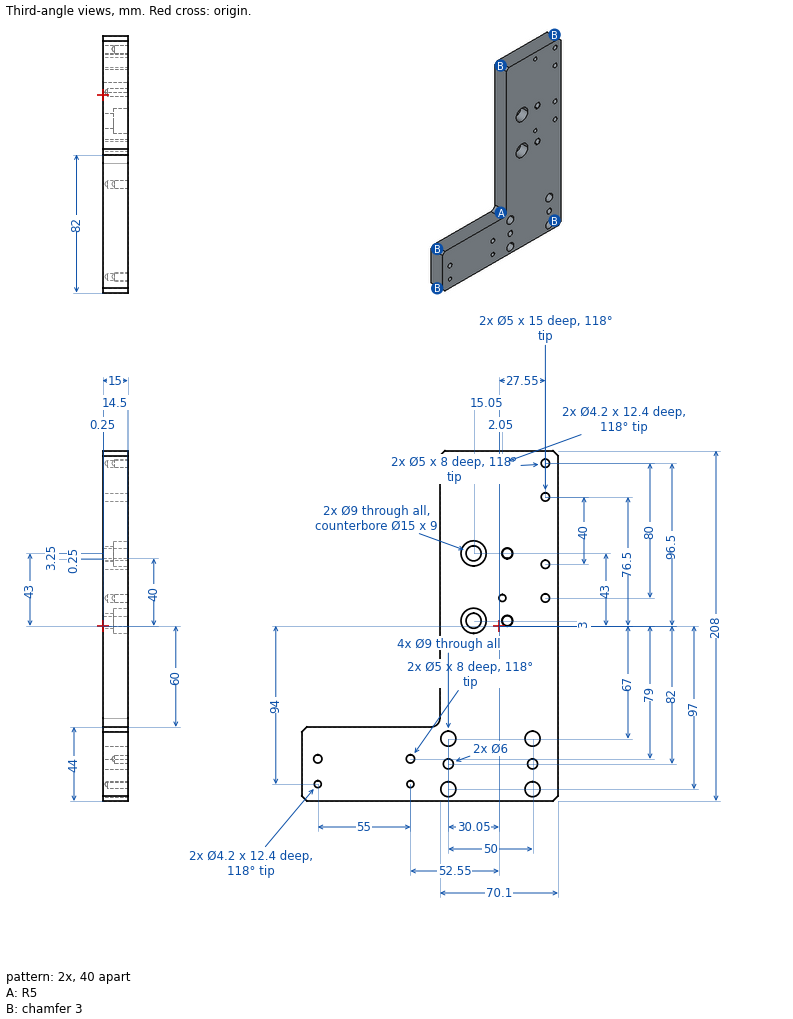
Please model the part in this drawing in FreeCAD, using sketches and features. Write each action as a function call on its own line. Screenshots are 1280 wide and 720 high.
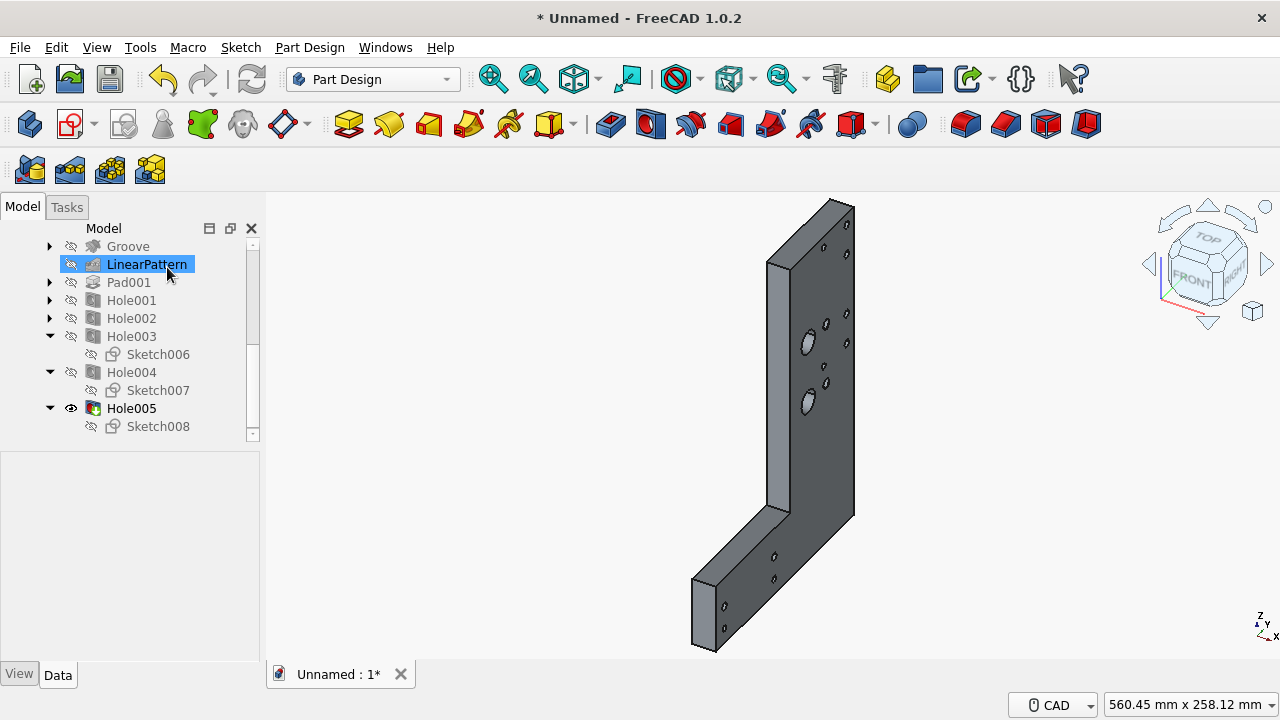
click(824, 477)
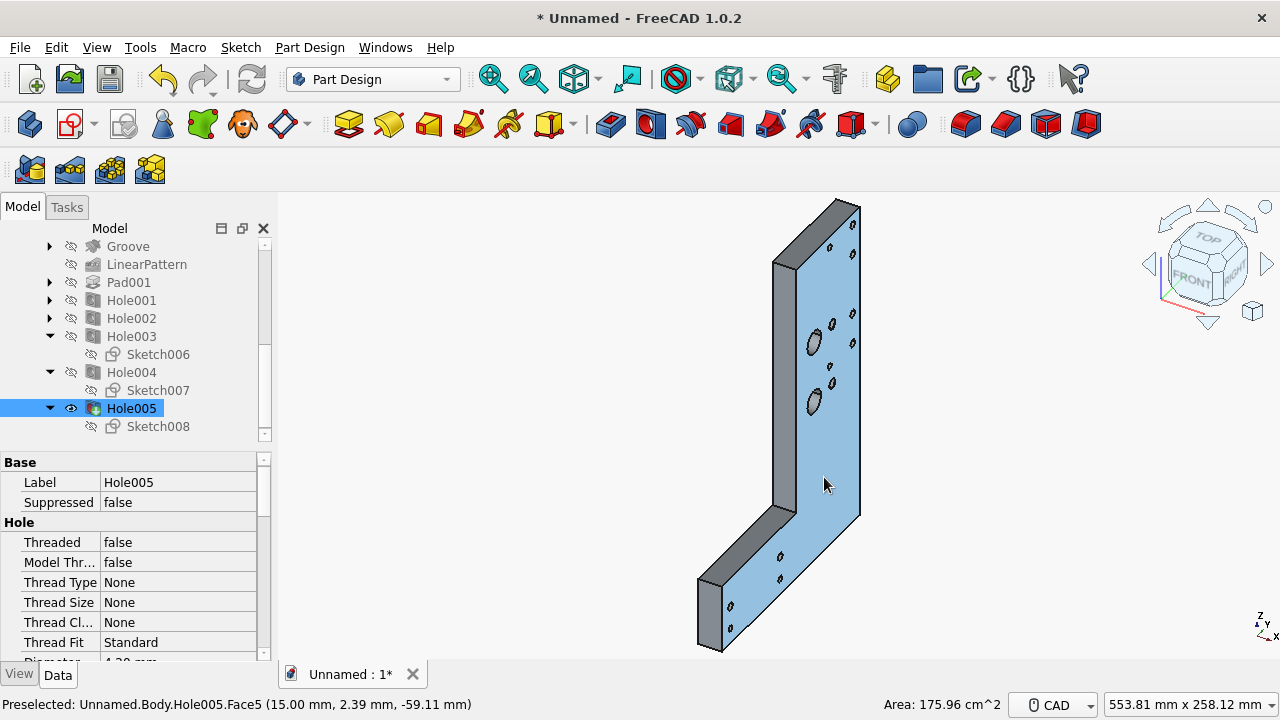
click(70, 124)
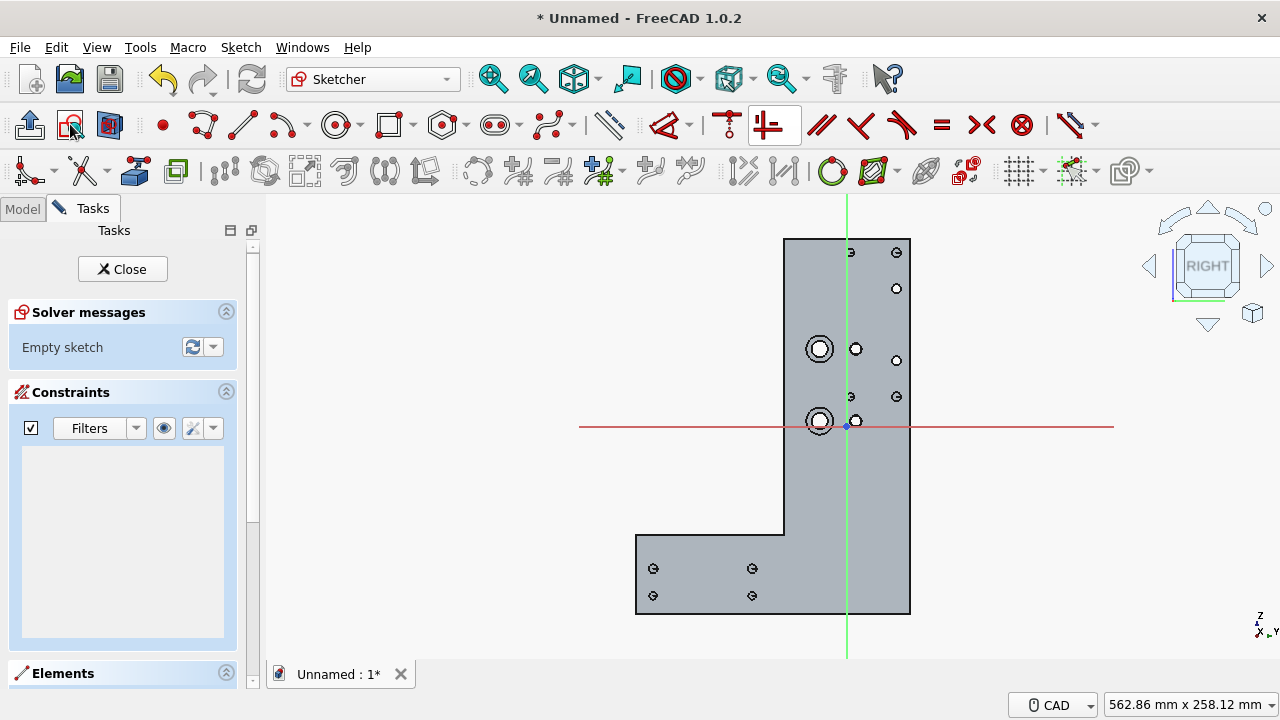
scroll(1109, 631, up, 2)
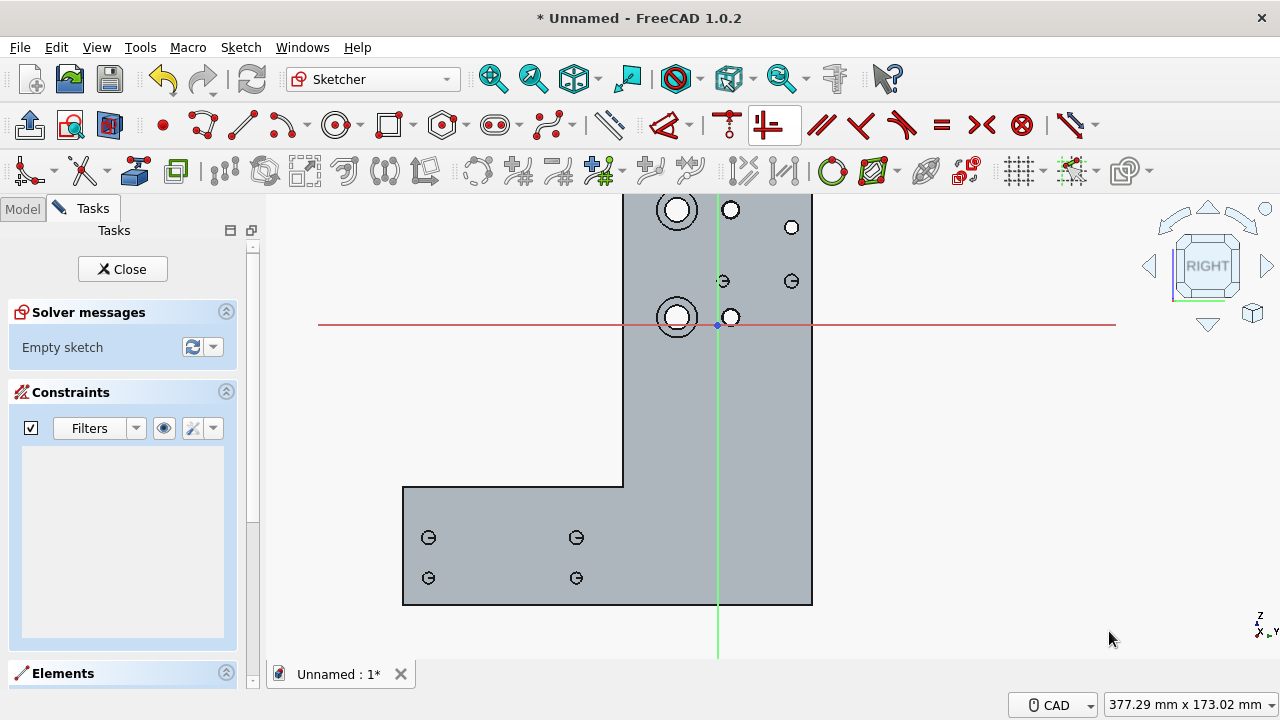
key(g)
key(c)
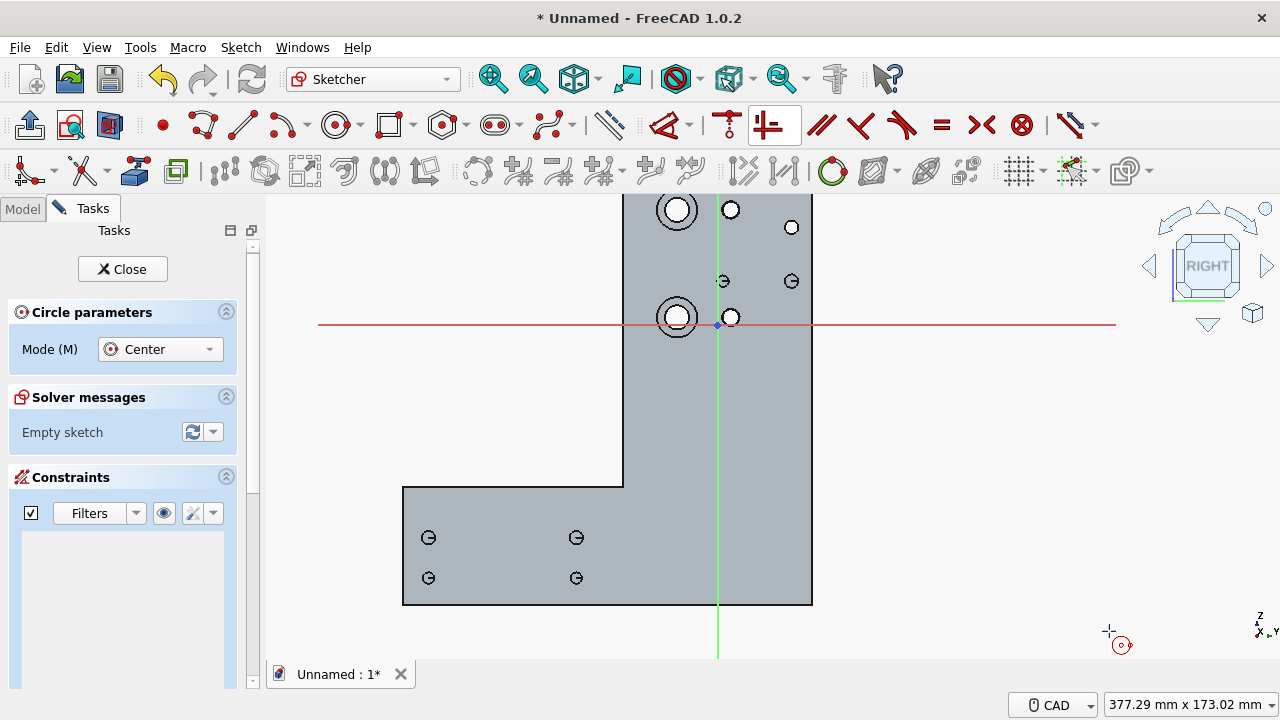
scroll(637, 506, up, 4)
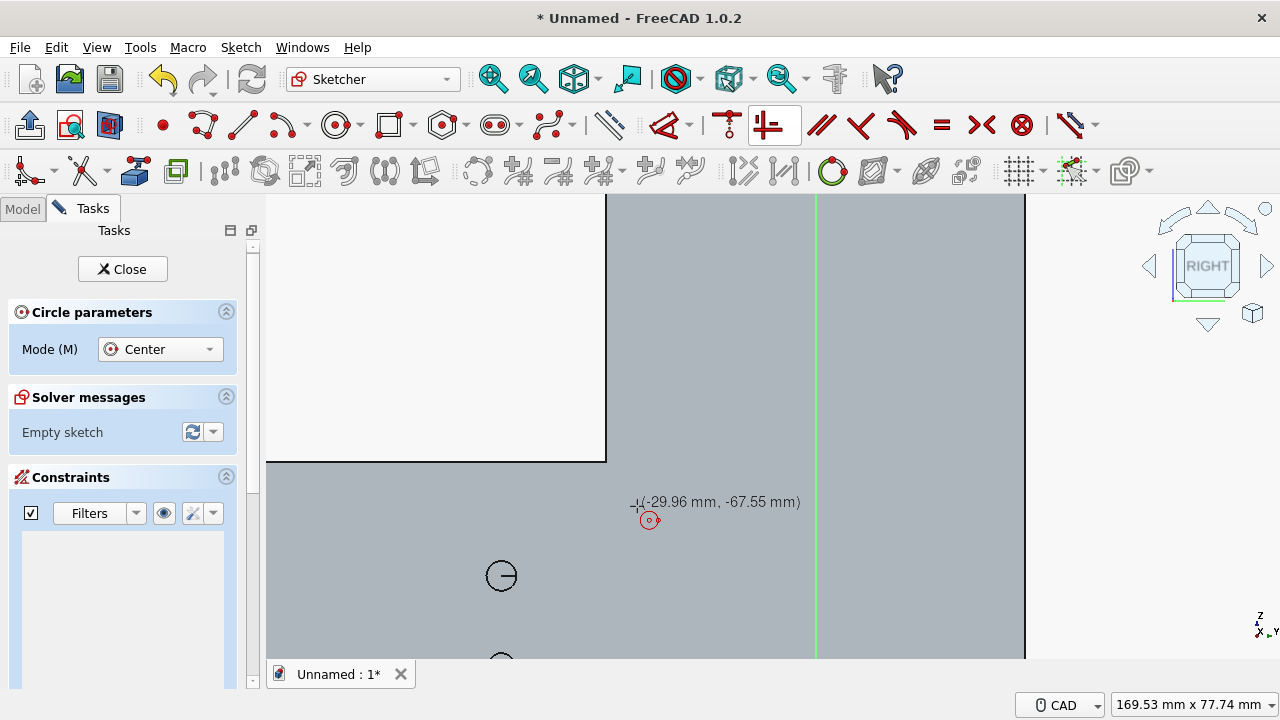
click(636, 504)
click(655, 485)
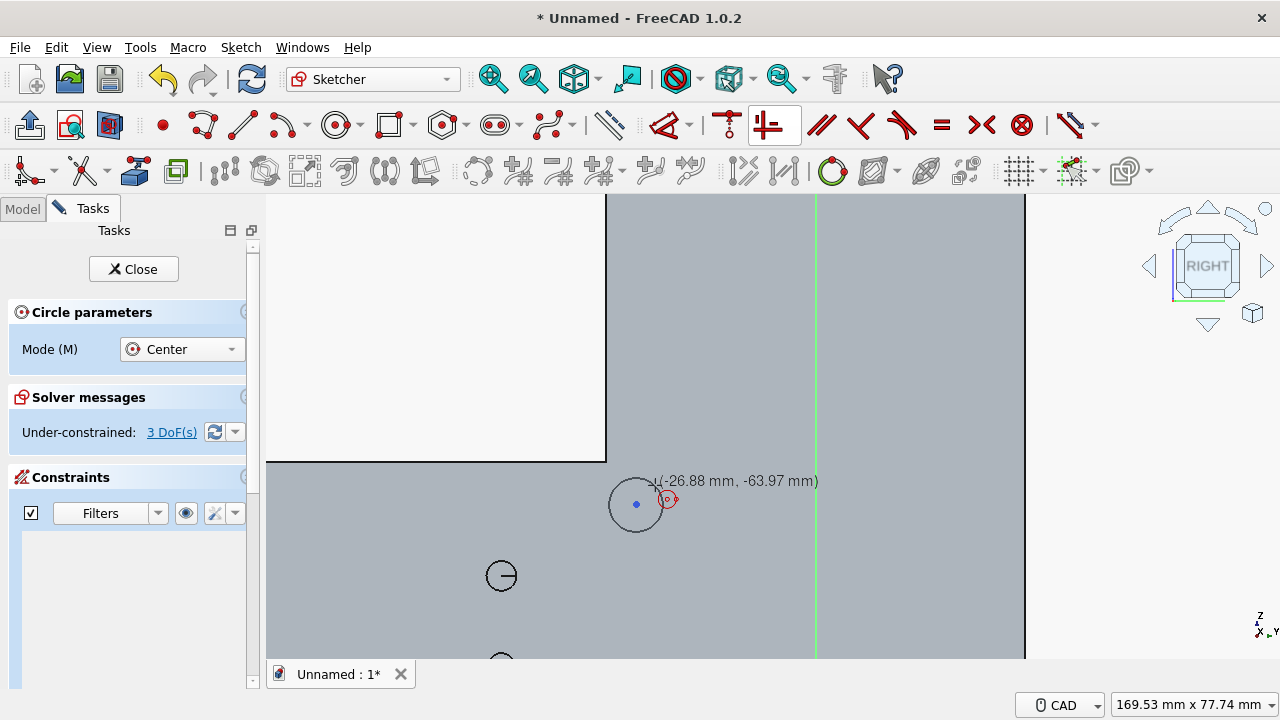
scroll(638, 442, down, 4)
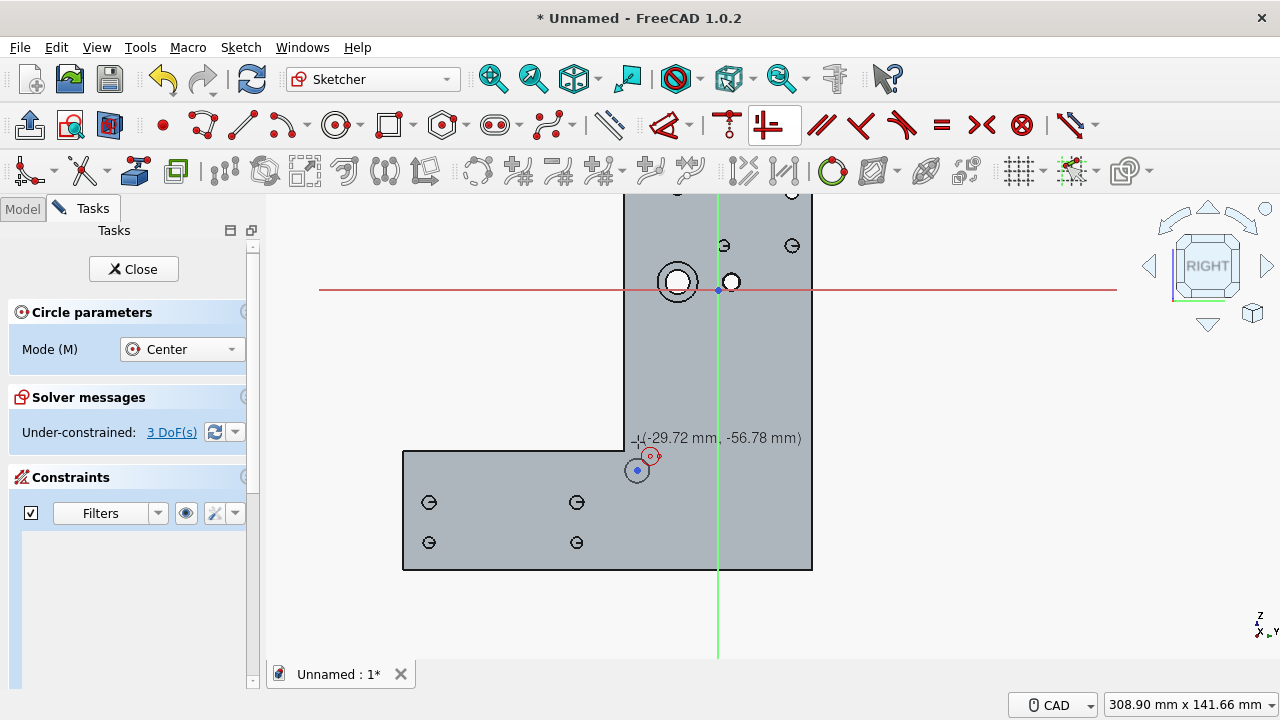
scroll(637, 551, up, 4)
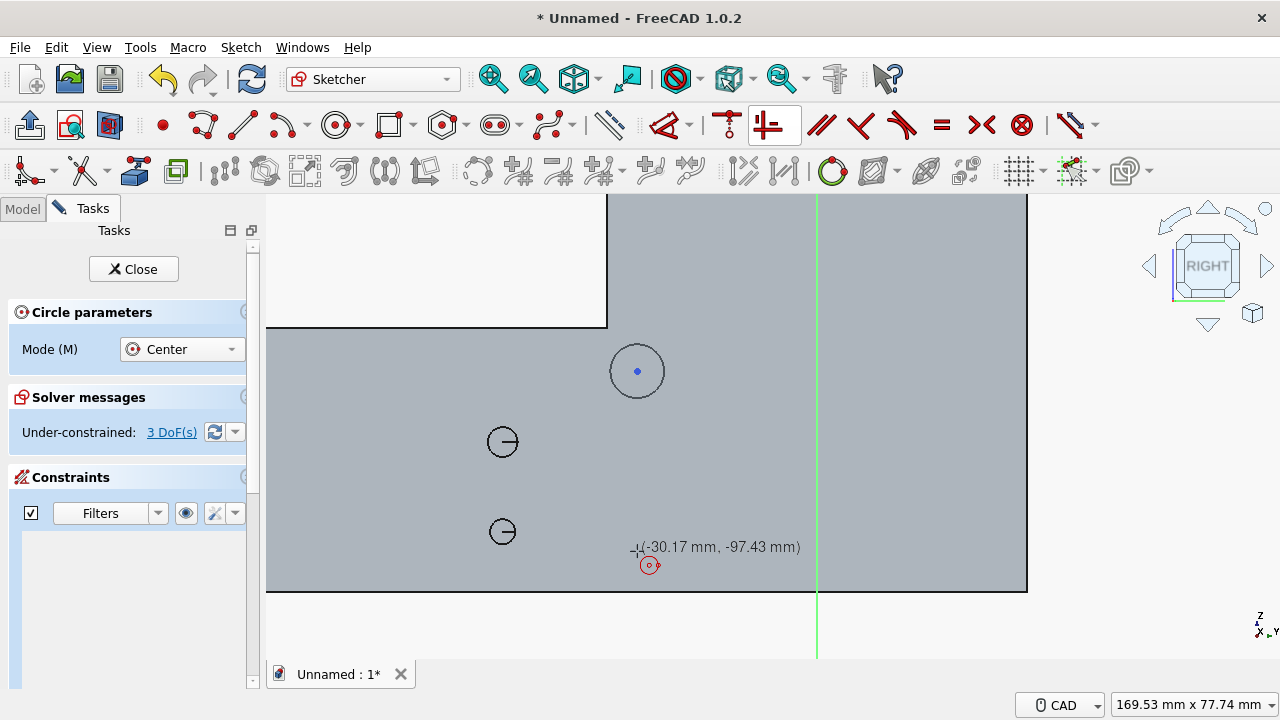
click(637, 550)
click(656, 531)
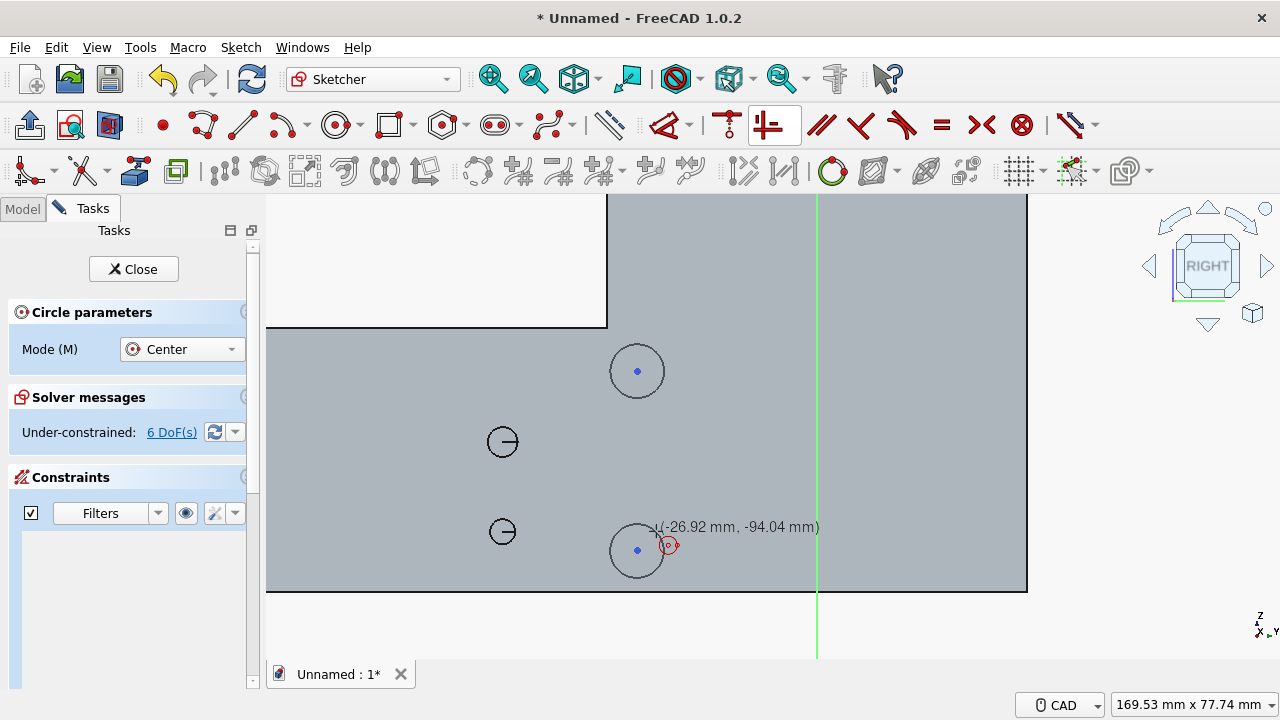
click(936, 370)
click(955, 351)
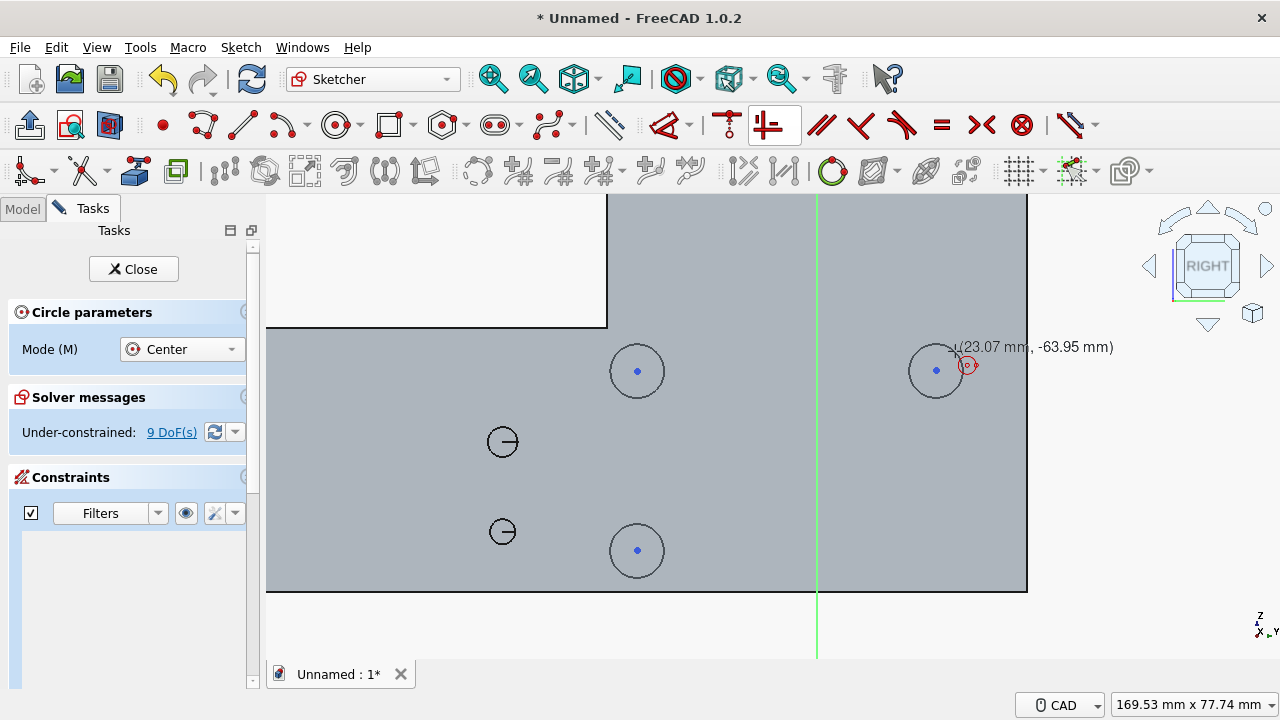
click(936, 550)
click(955, 531)
key(Escape)